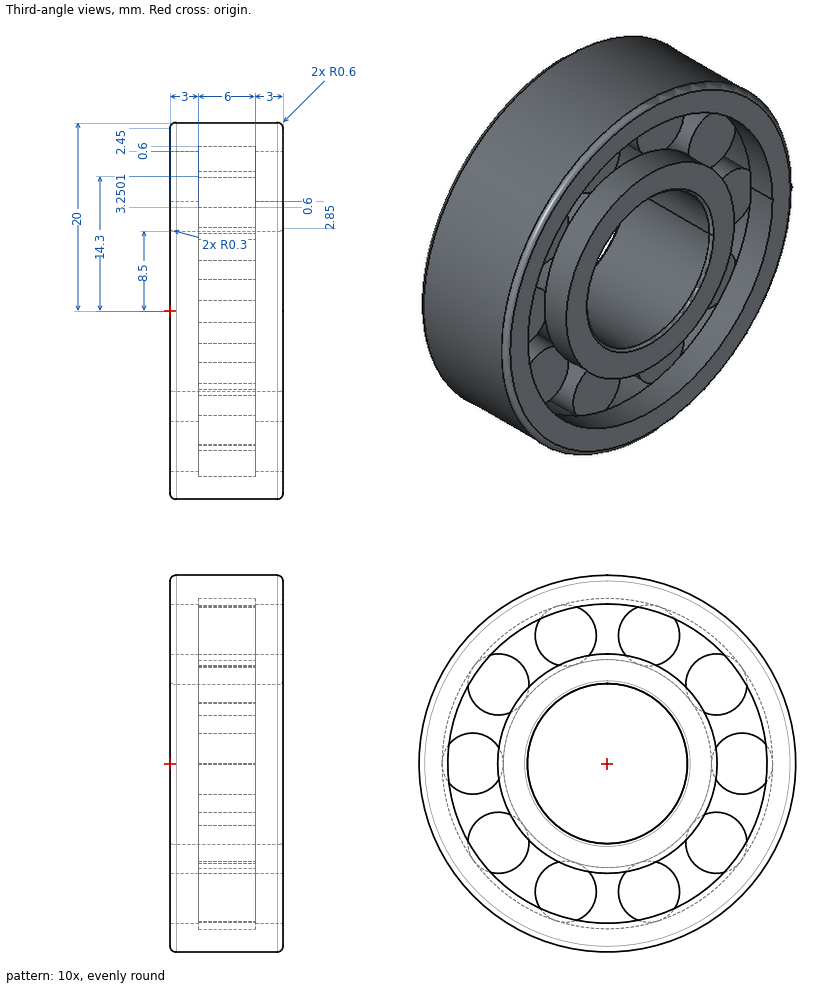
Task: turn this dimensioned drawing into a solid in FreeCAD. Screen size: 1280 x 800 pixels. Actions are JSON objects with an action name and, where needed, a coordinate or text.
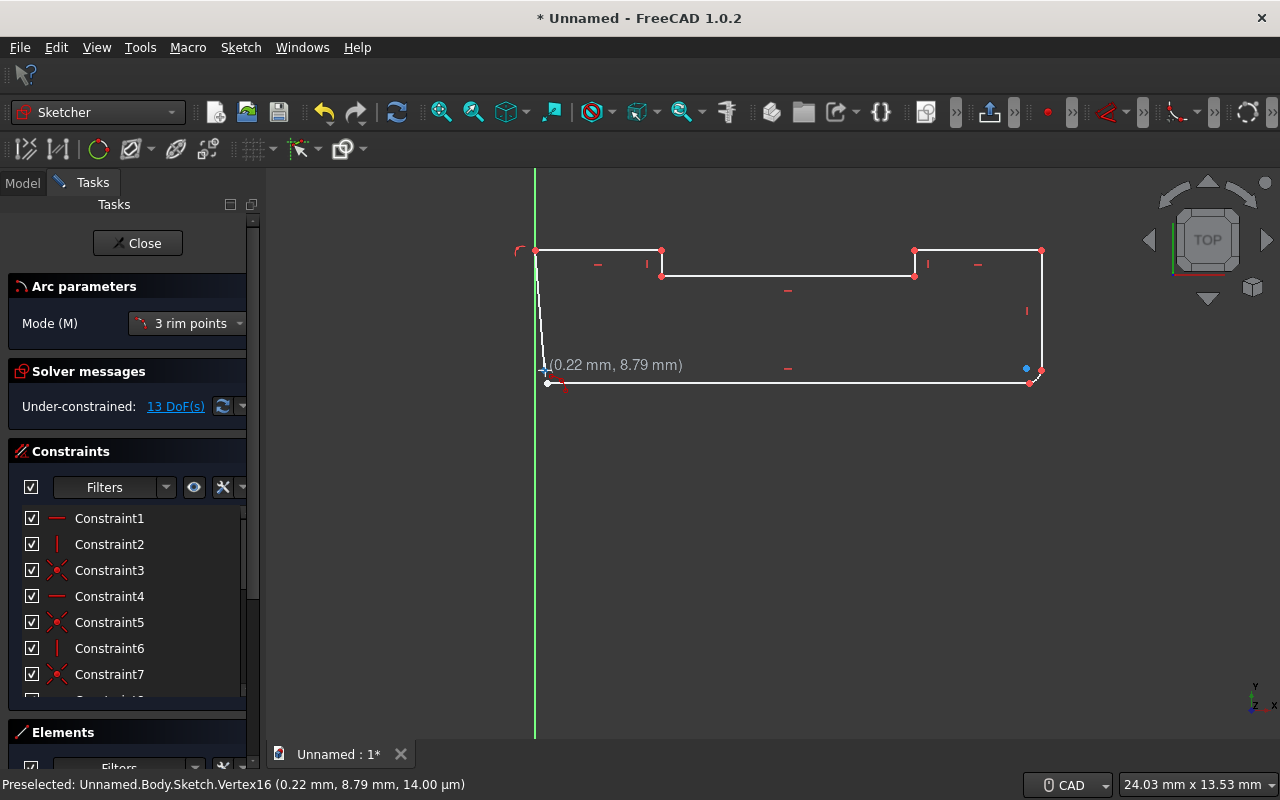
{"action": "scroll", "coordinate": [548, 382], "scroll_direction": "up", "scroll_amount": 2}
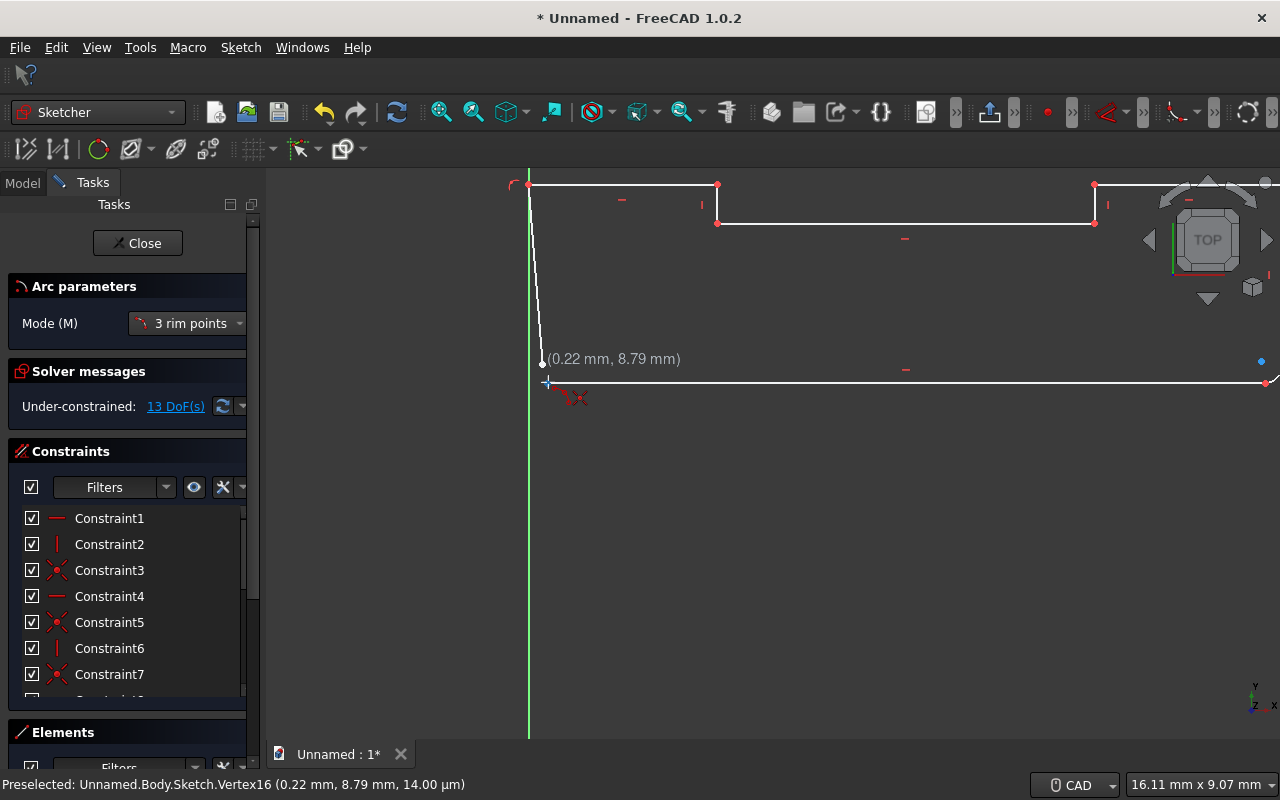
{"action": "left_click", "coordinate": [548, 383]}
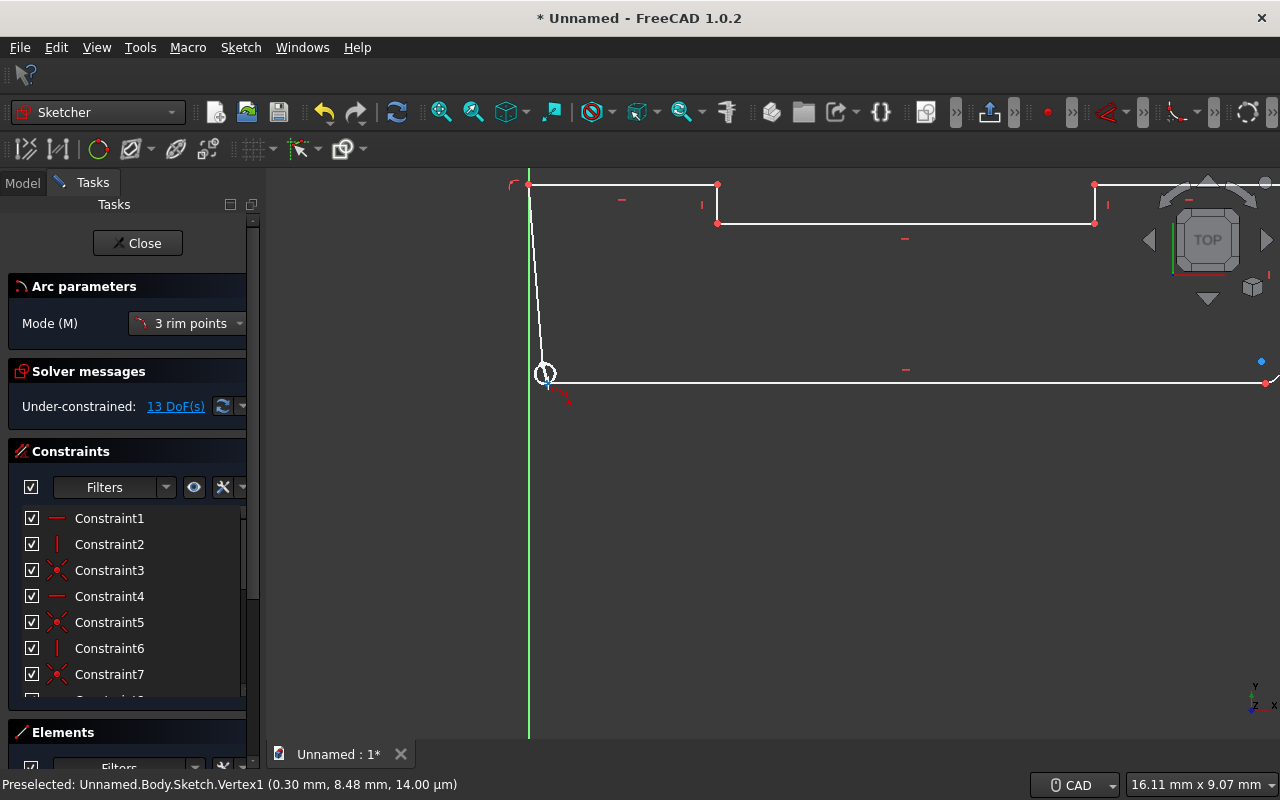
{"action": "scroll", "coordinate": [534, 377], "scroll_direction": "up", "scroll_amount": 6}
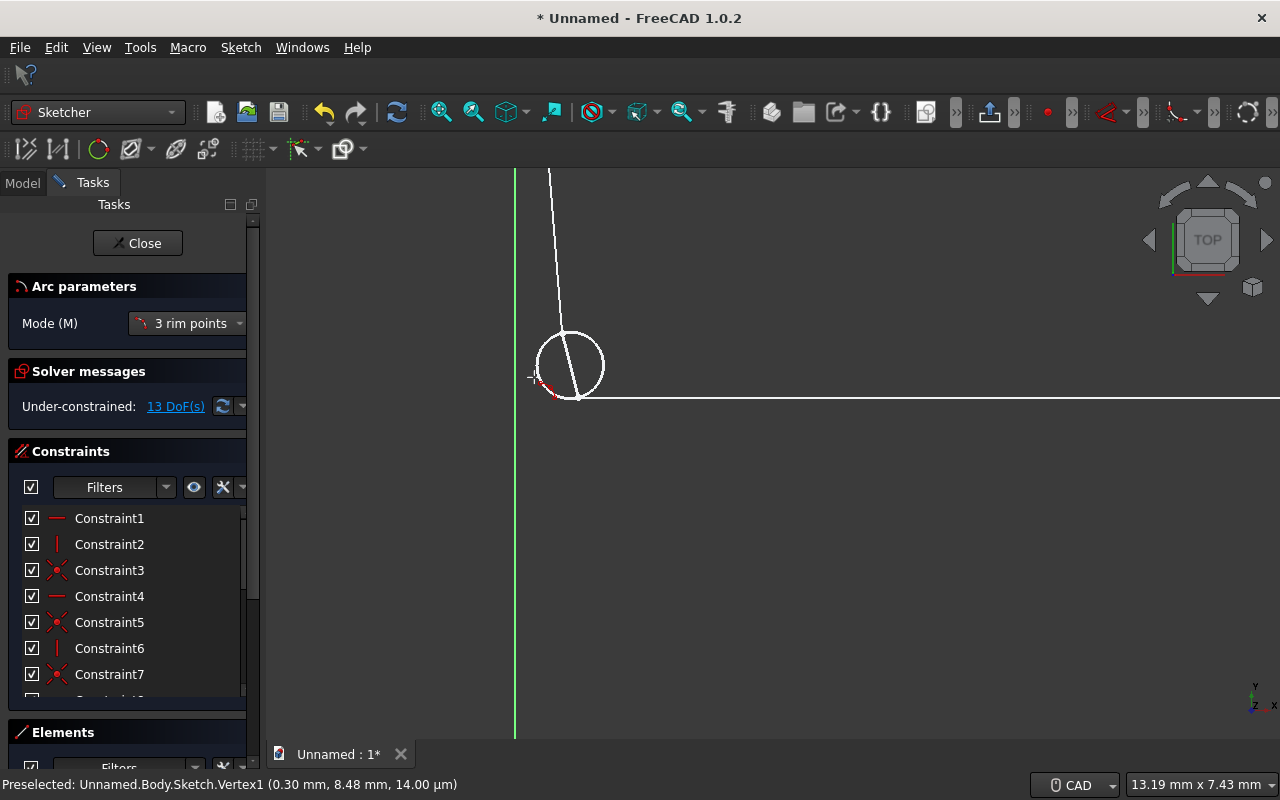
{"action": "left_click", "coordinate": [534, 375]}
{"action": "key", "text": "Escape"}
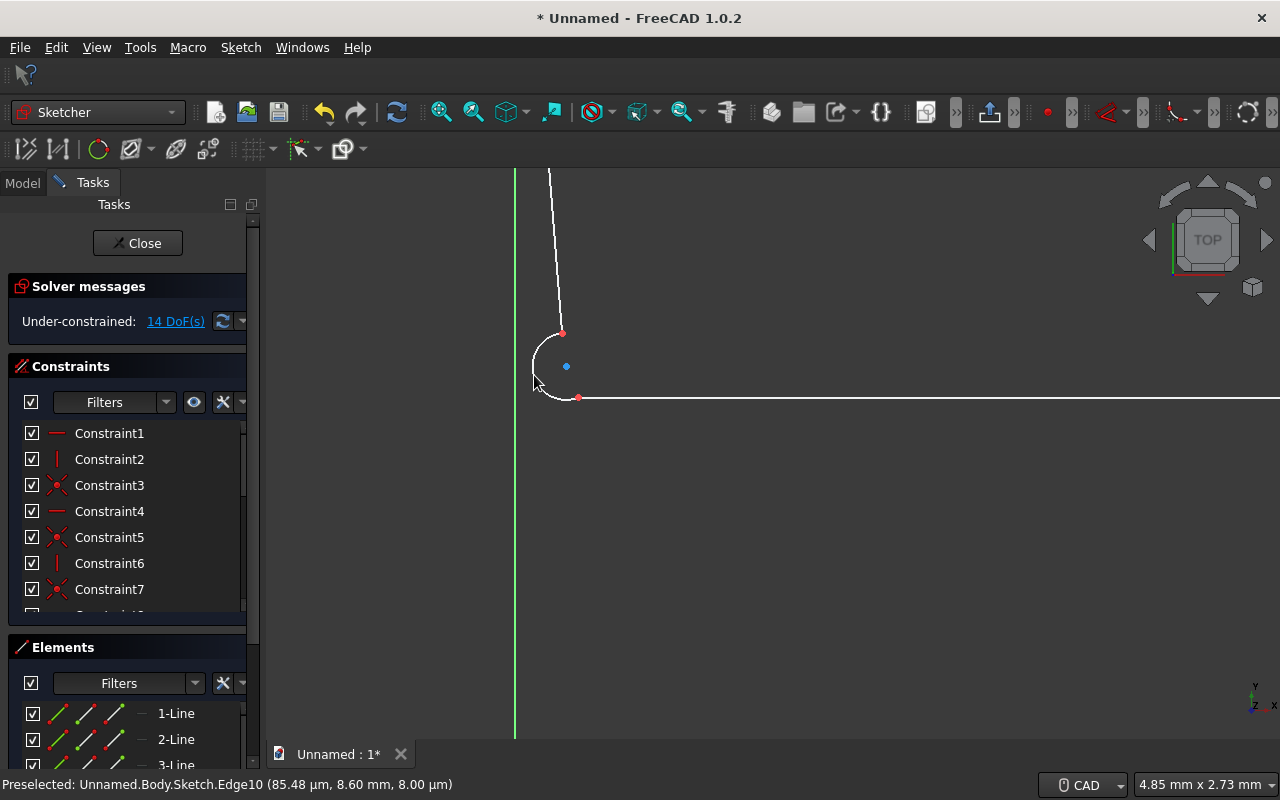
{"action": "scroll", "coordinate": [538, 375], "scroll_direction": "down", "scroll_amount": 10}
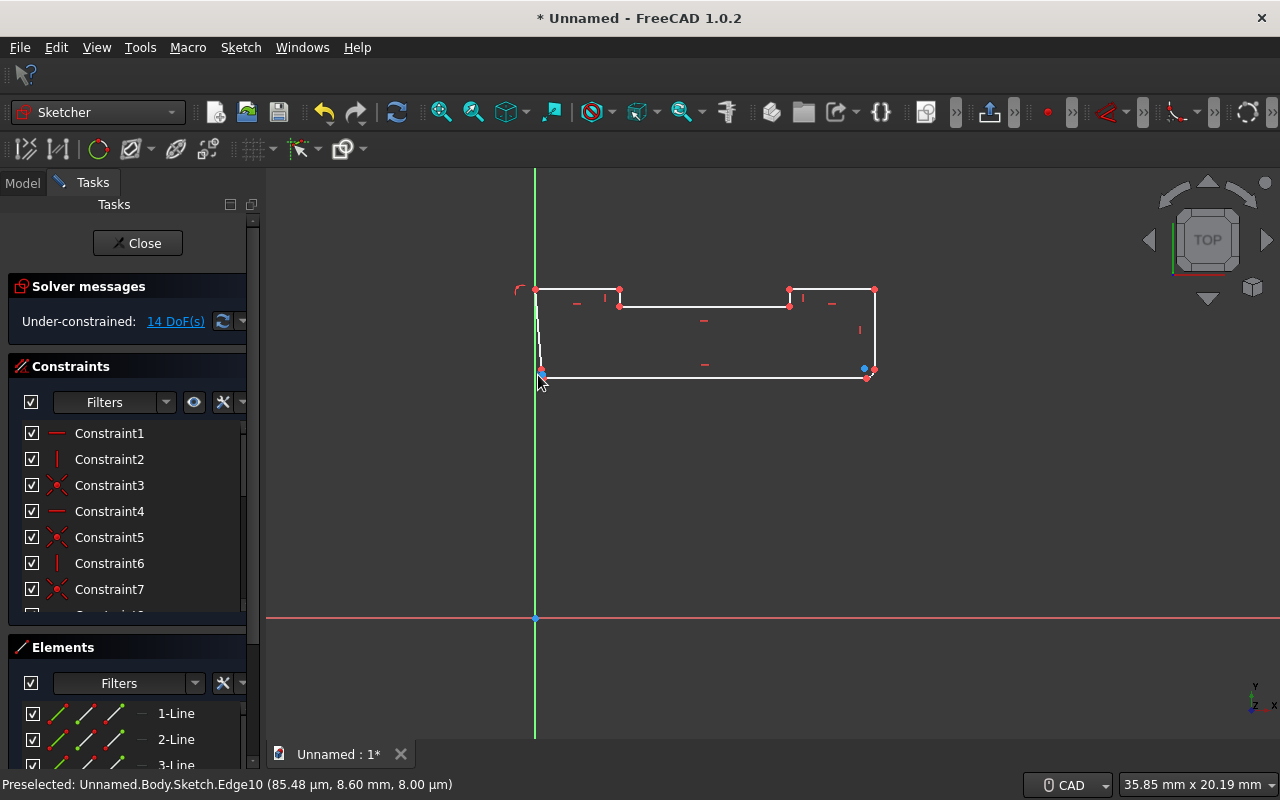
{"action": "left_click", "coordinate": [608, 378]}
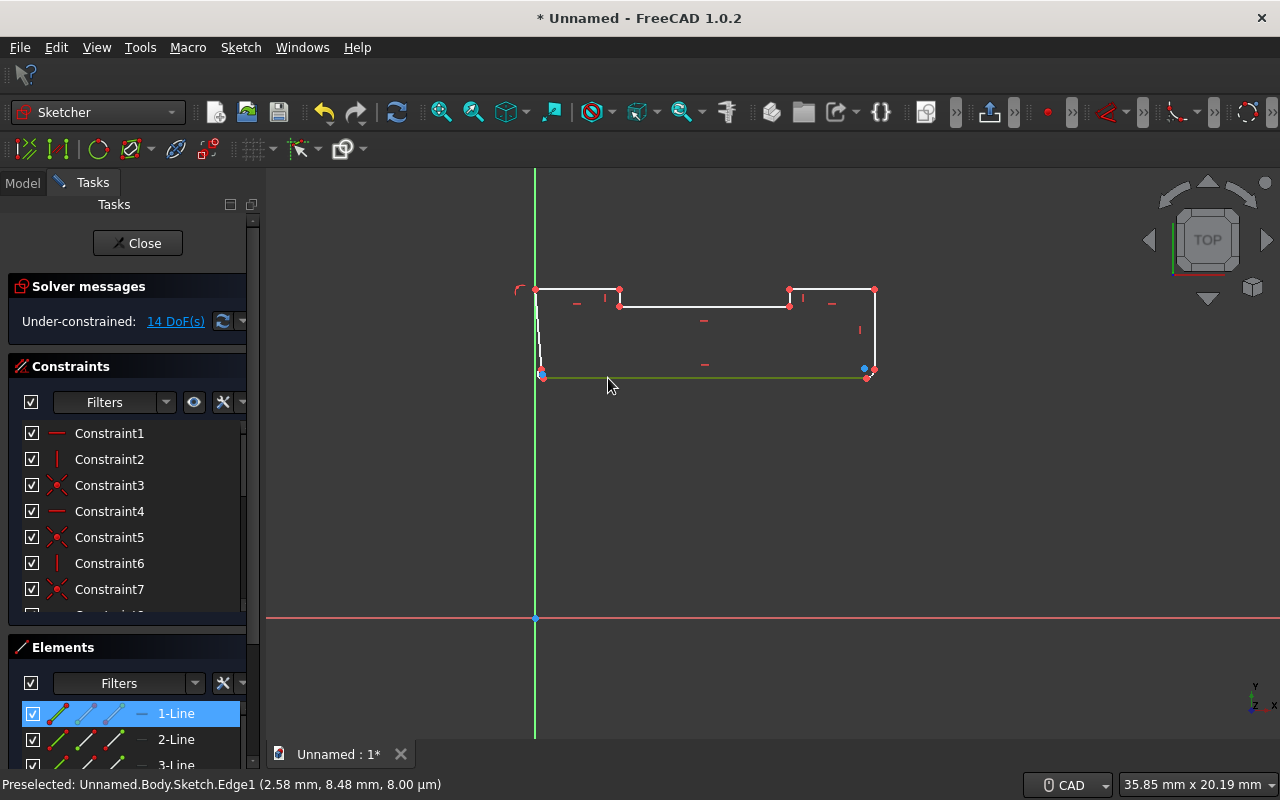
{"action": "scroll", "coordinate": [872, 375], "scroll_direction": "up", "scroll_amount": 4}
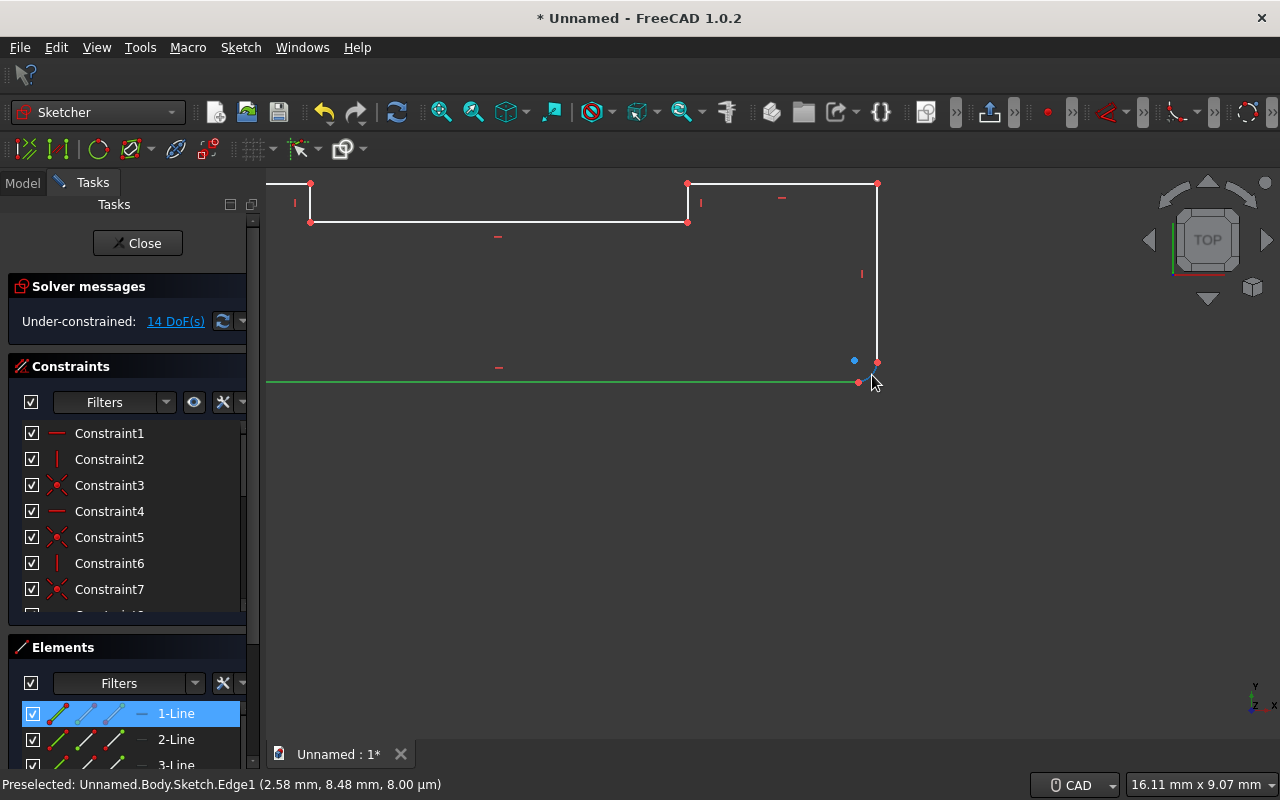
{"action": "left_click", "coordinate": [871, 375]}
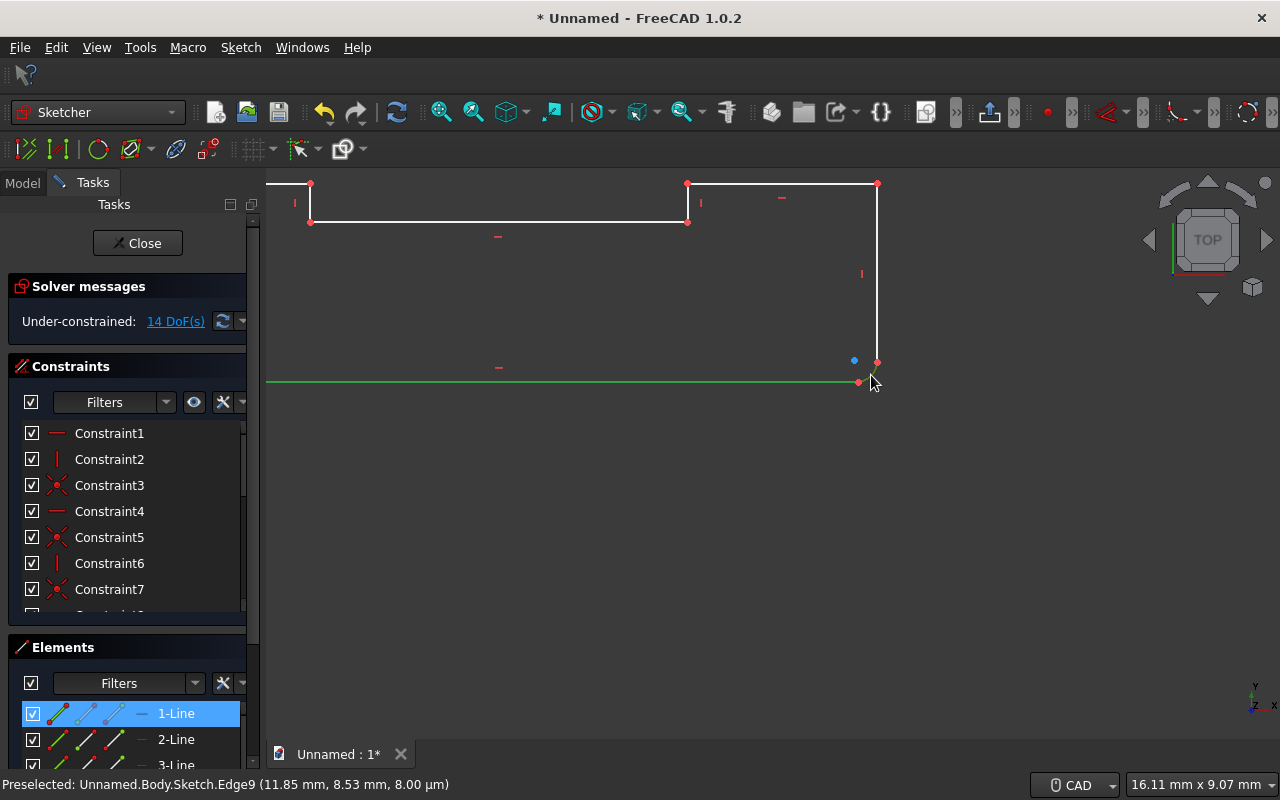
{"action": "key", "text": "t"}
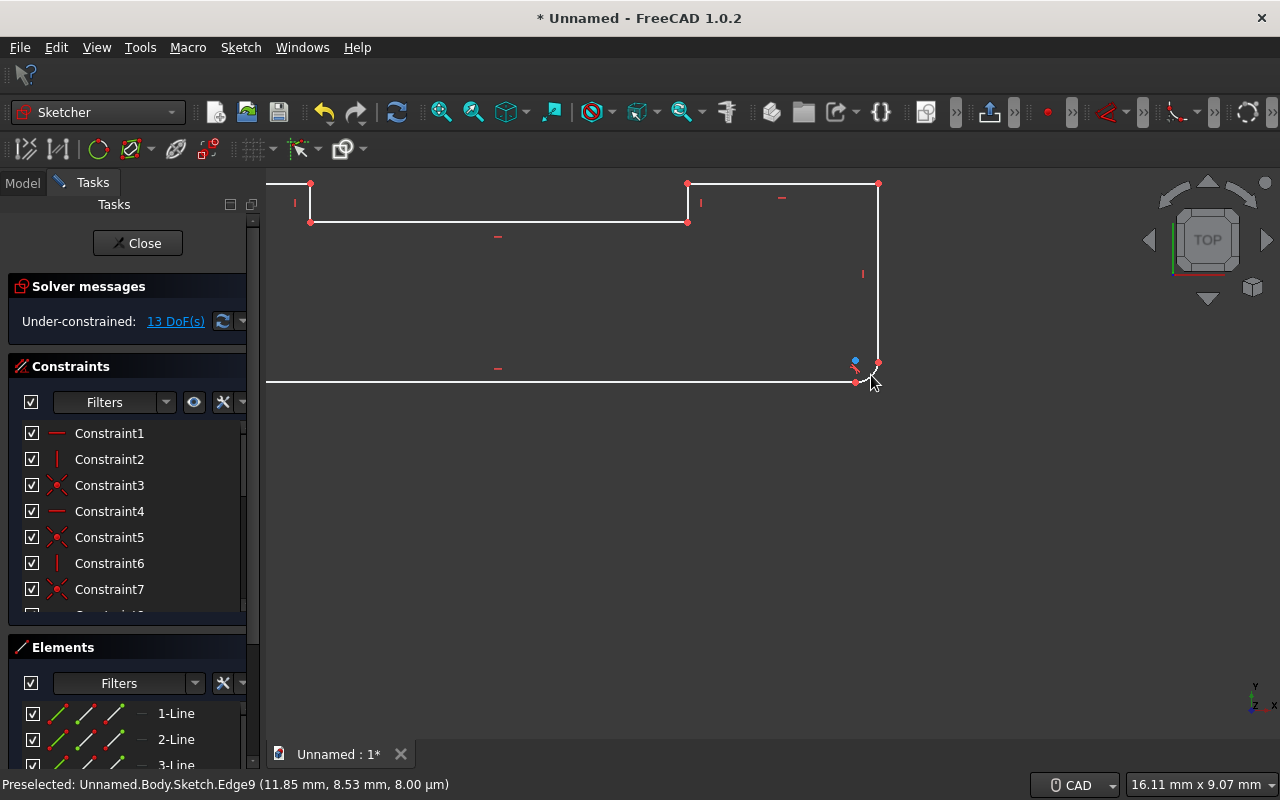
{"action": "left_click", "coordinate": [355, 382]}